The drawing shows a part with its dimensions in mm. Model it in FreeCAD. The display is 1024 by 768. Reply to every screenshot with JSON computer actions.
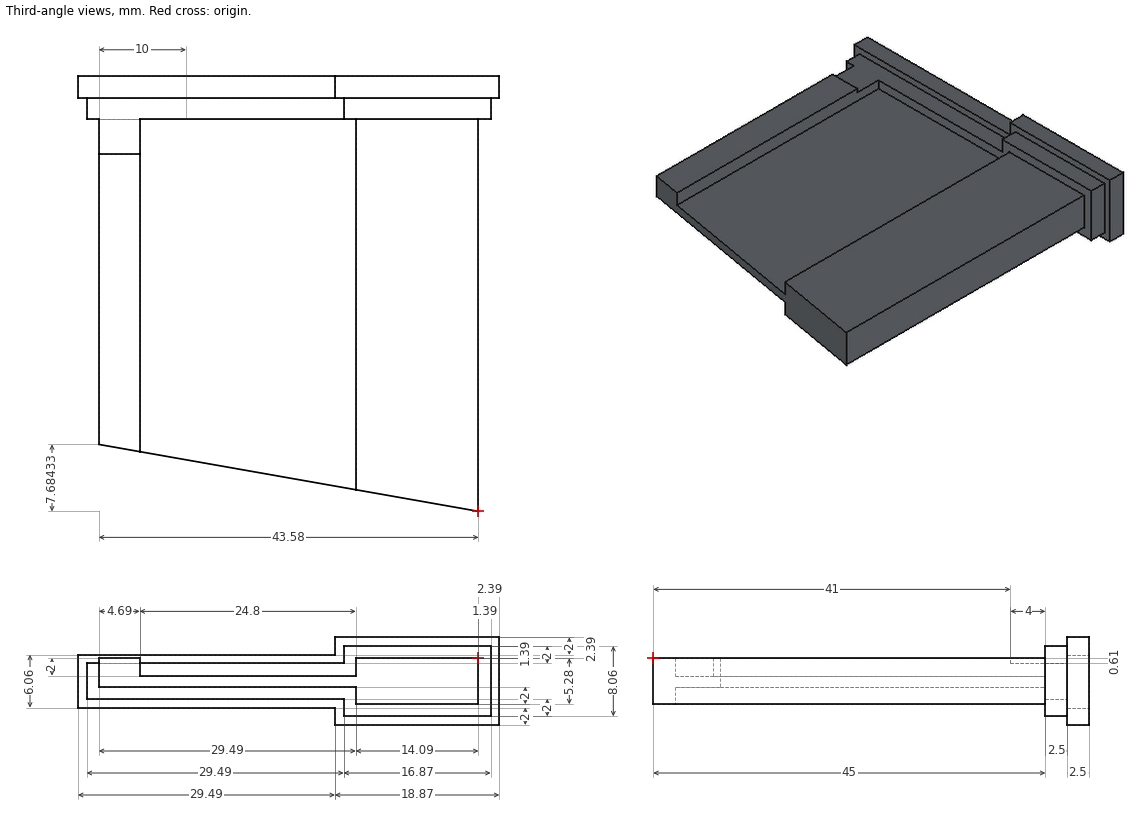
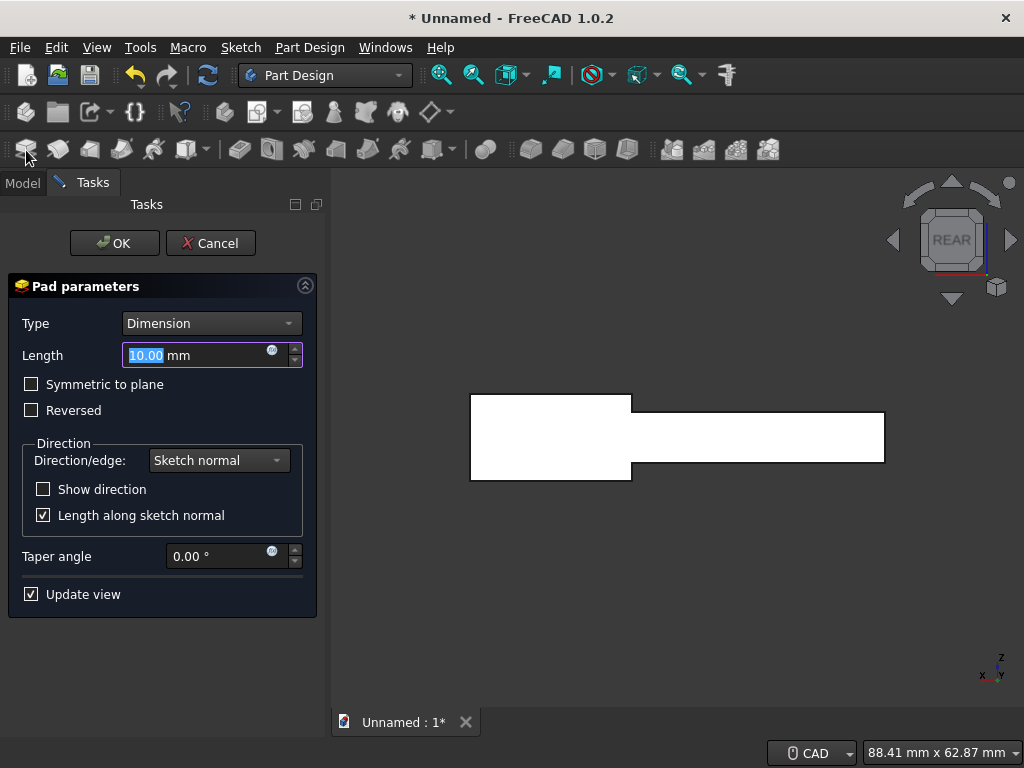
{"action": "type", "text": "2.5"}
{"action": "key", "text": "Tab"}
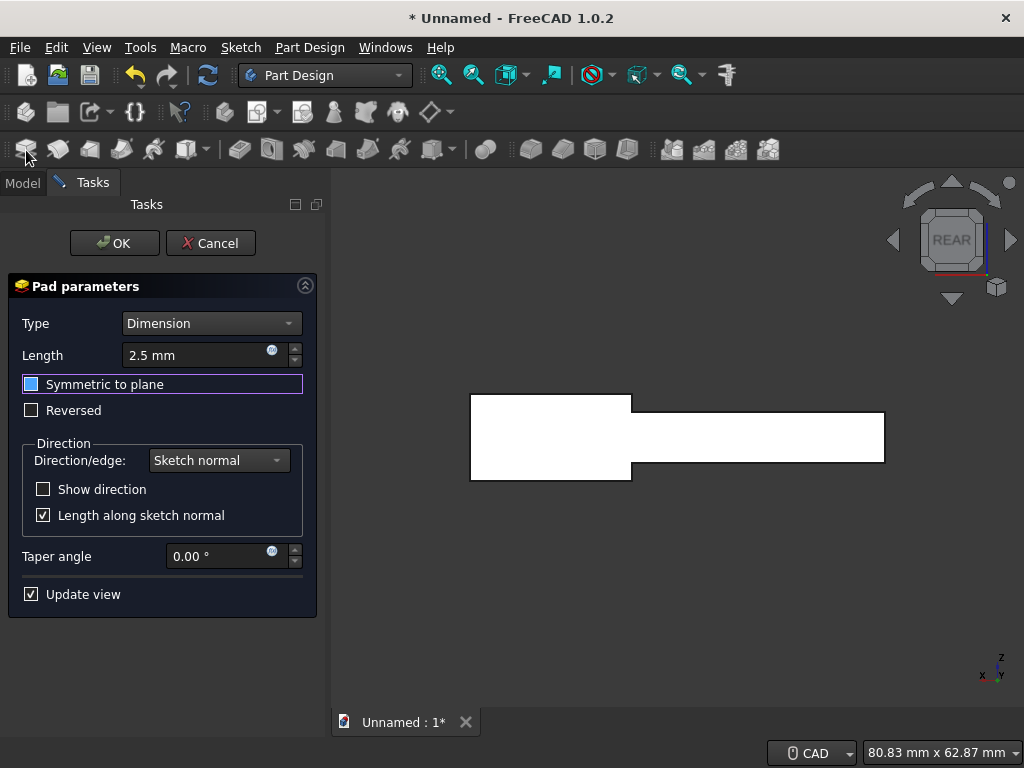
{"action": "left_click", "coordinate": [115, 243]}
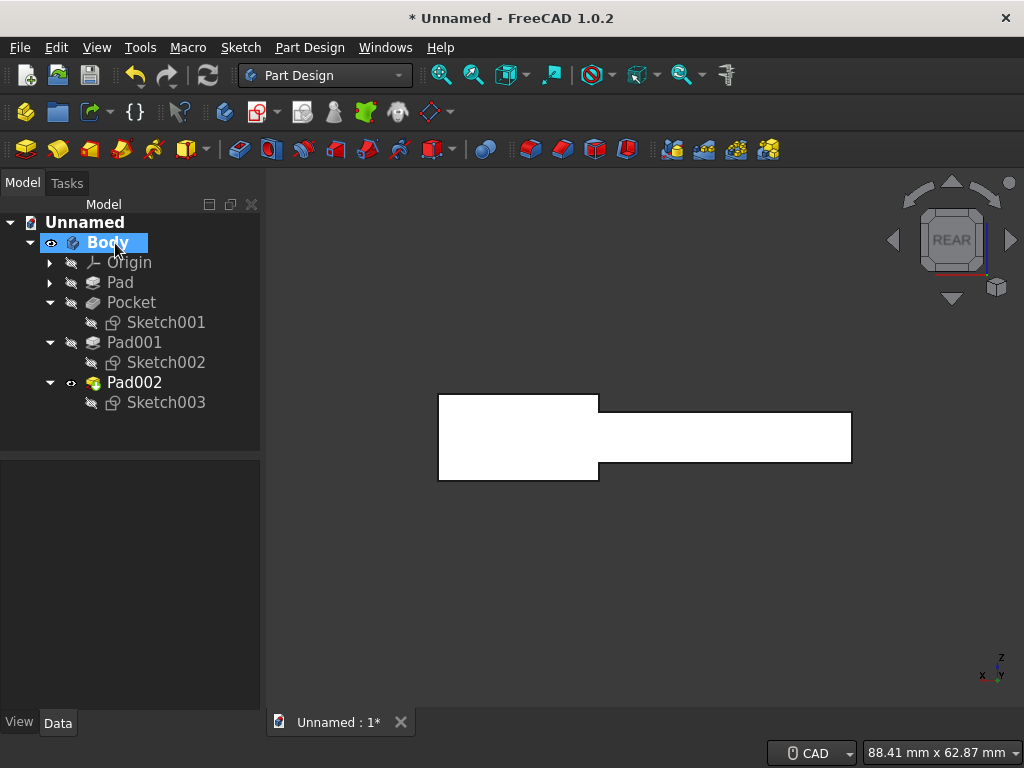
{"action": "key", "text": "6"}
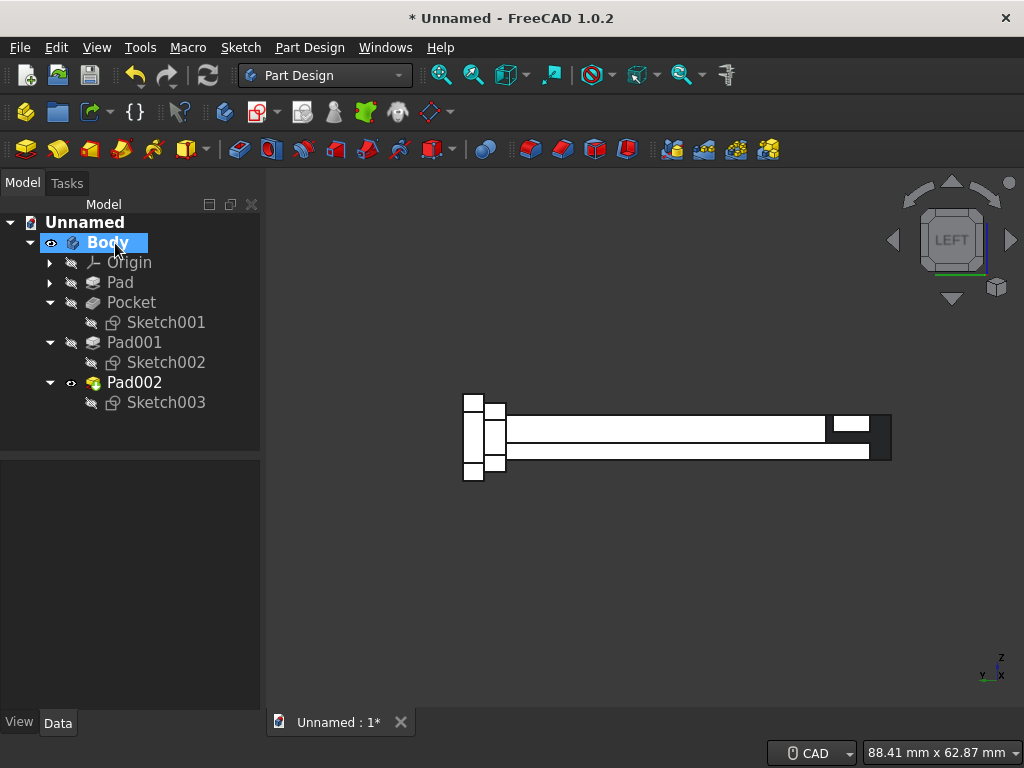
{"action": "left_click", "coordinate": [529, 428]}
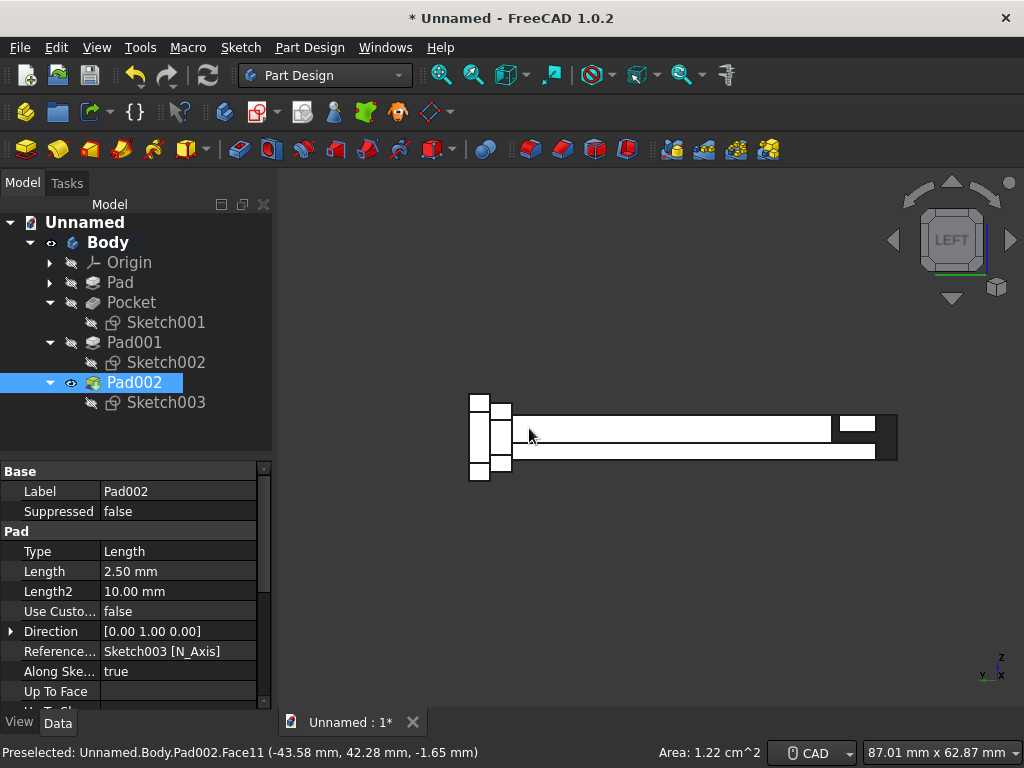
{"action": "left_click", "coordinate": [258, 112]}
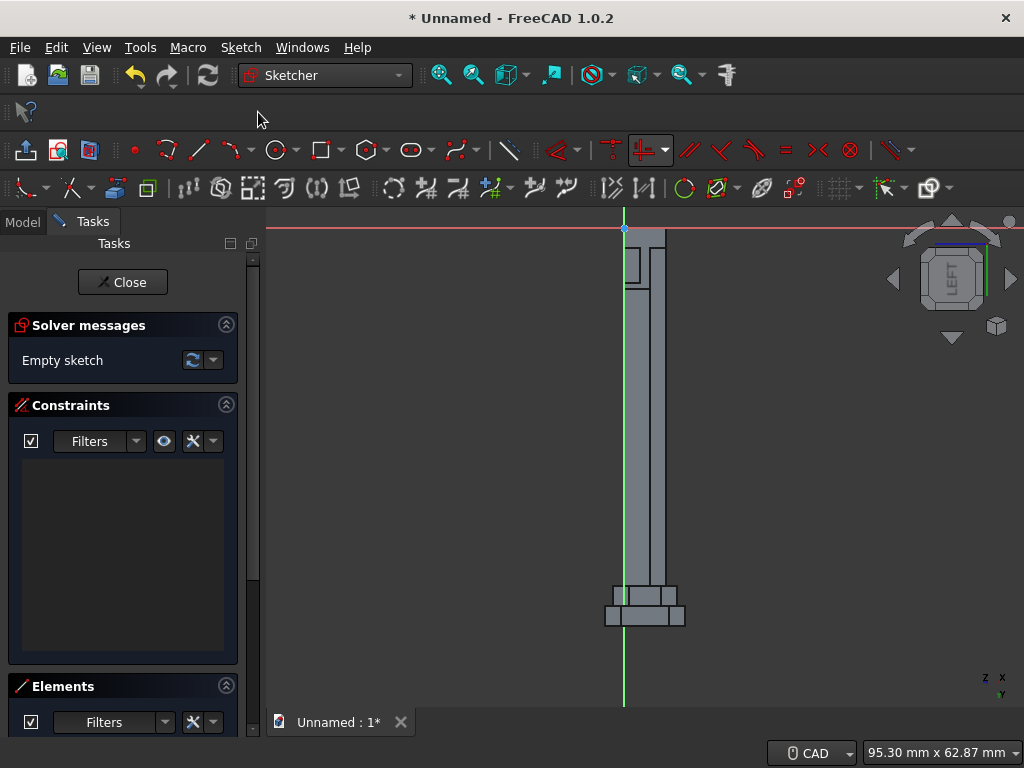
{"action": "key", "text": "q s"}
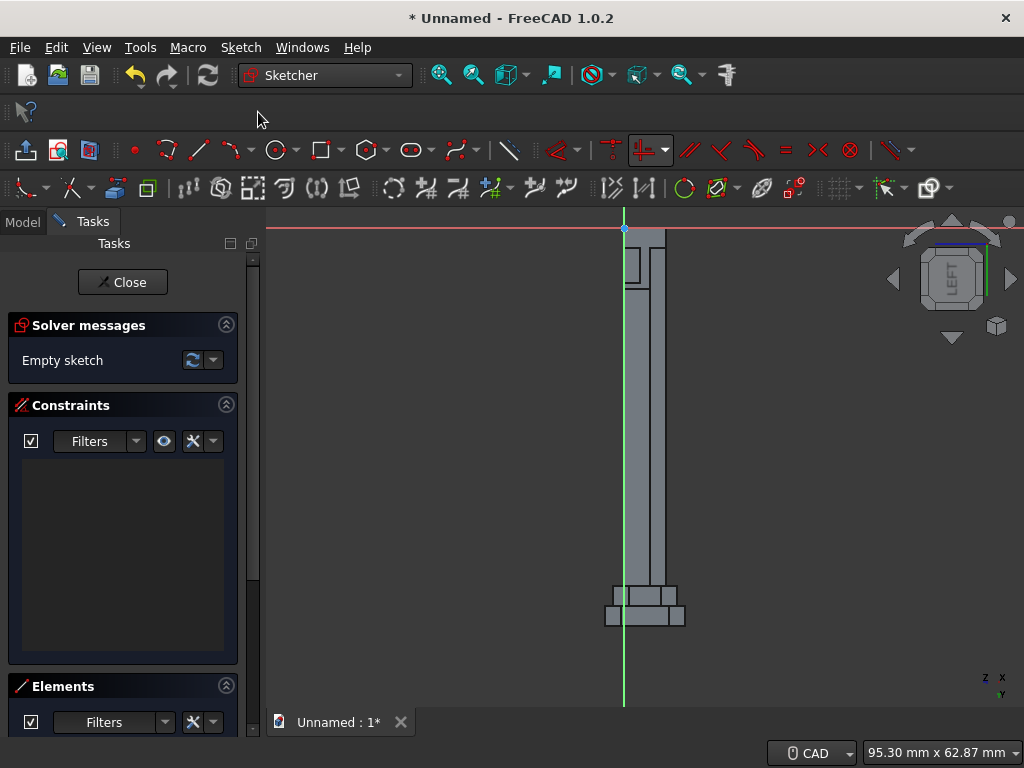
{"action": "scroll", "coordinate": [633, 584], "scroll_direction": "up", "scroll_amount": 11}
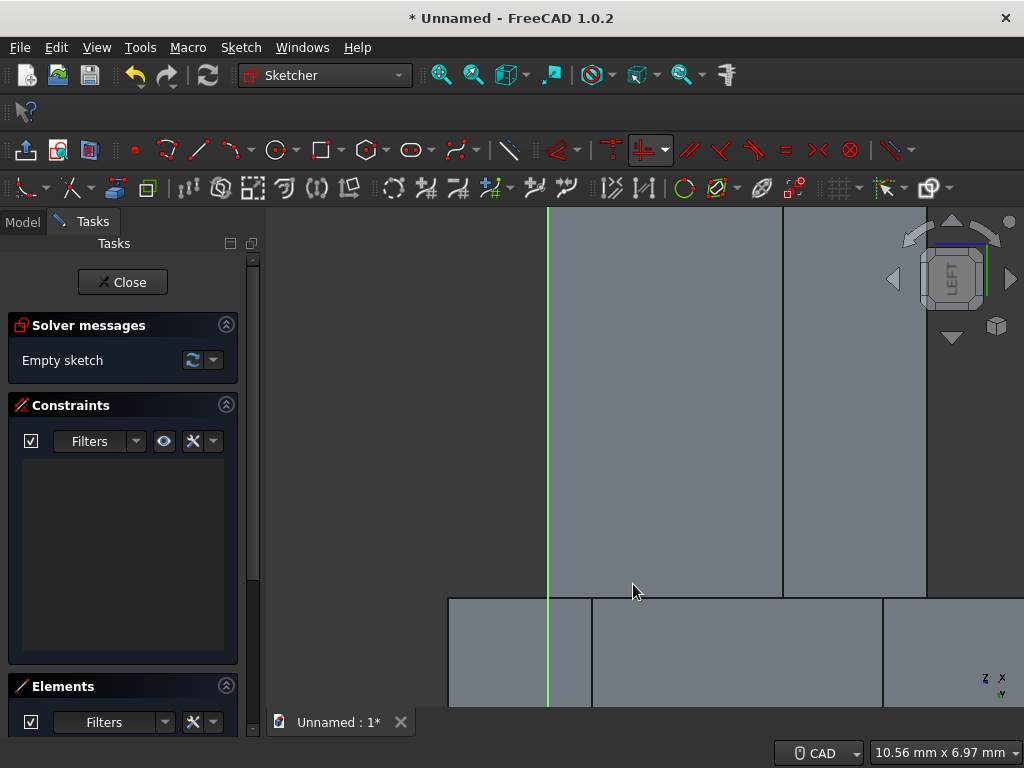
{"action": "key", "text": "g r"}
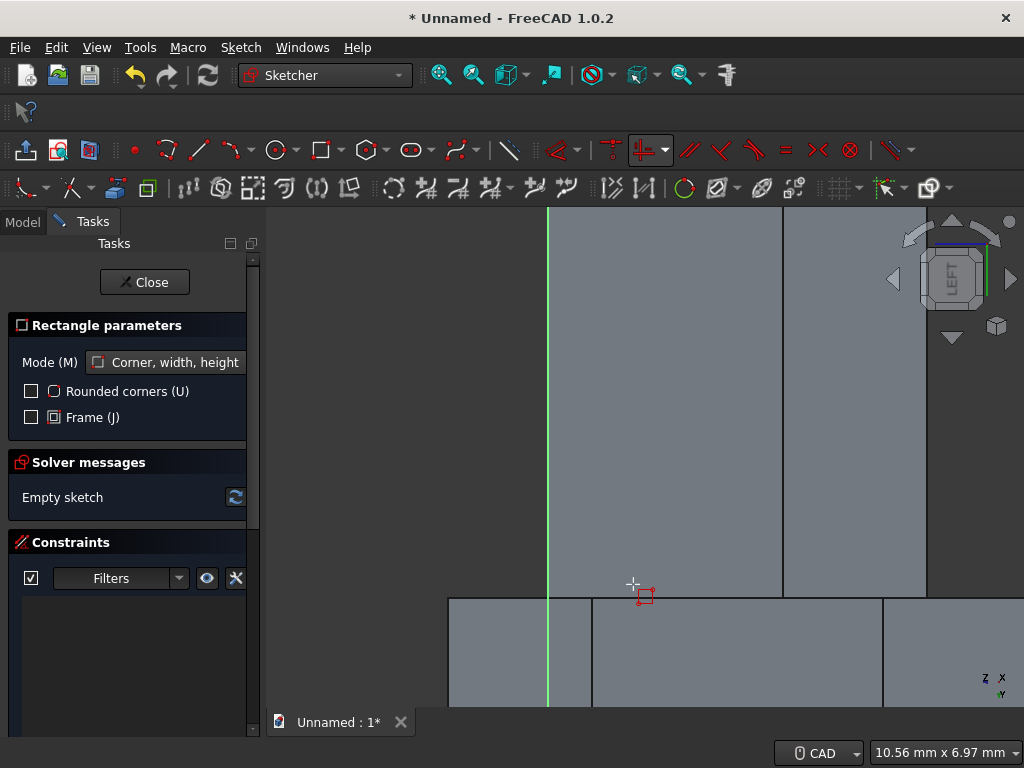
{"action": "left_click", "coordinate": [548, 311]}
{"action": "left_click", "coordinate": [592, 598]}
{"action": "key", "text": "Escape"}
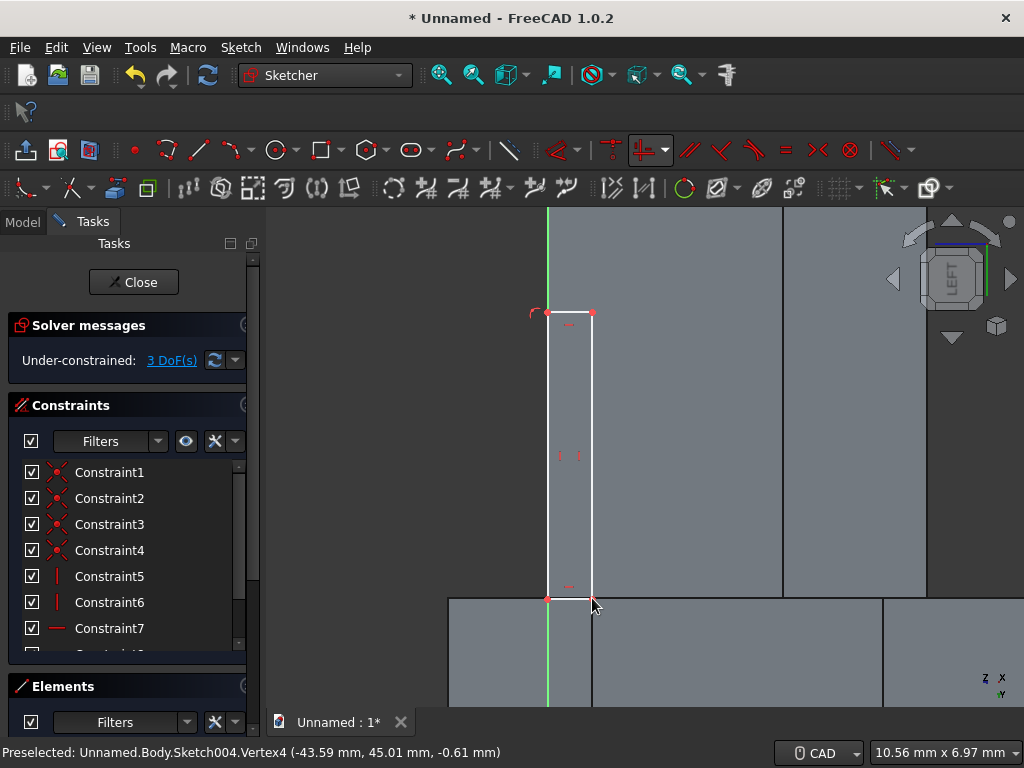
{"action": "key", "text": "d"}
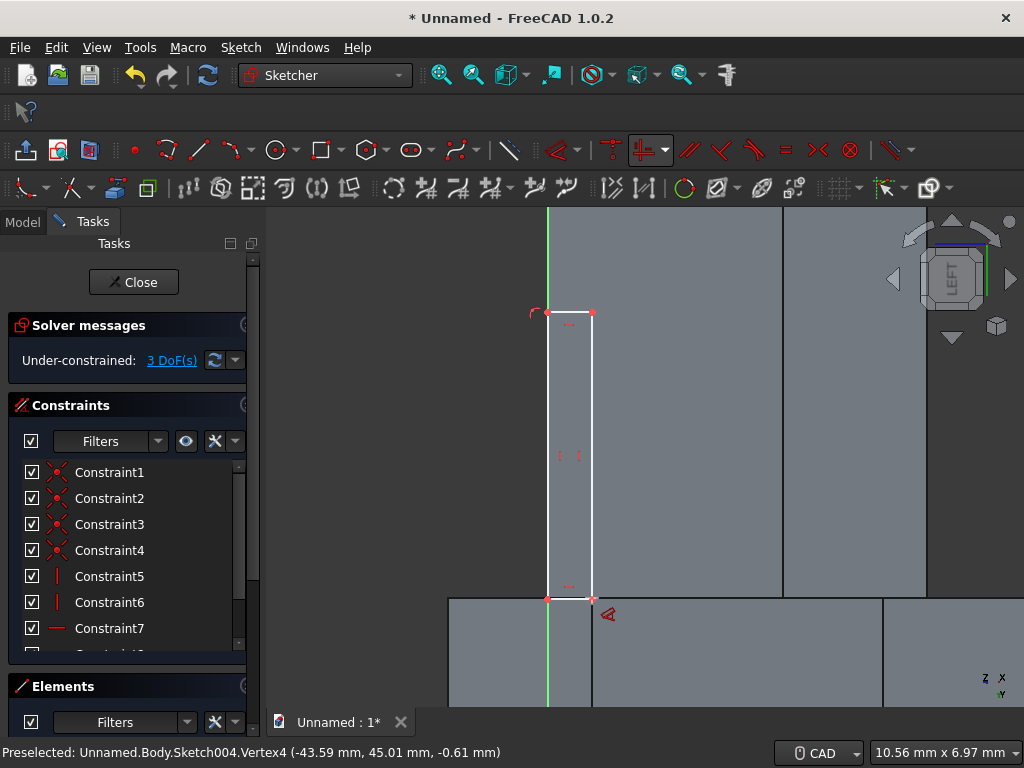
{"action": "left_click", "coordinate": [548, 398]}
{"action": "left_click", "coordinate": [514, 455]}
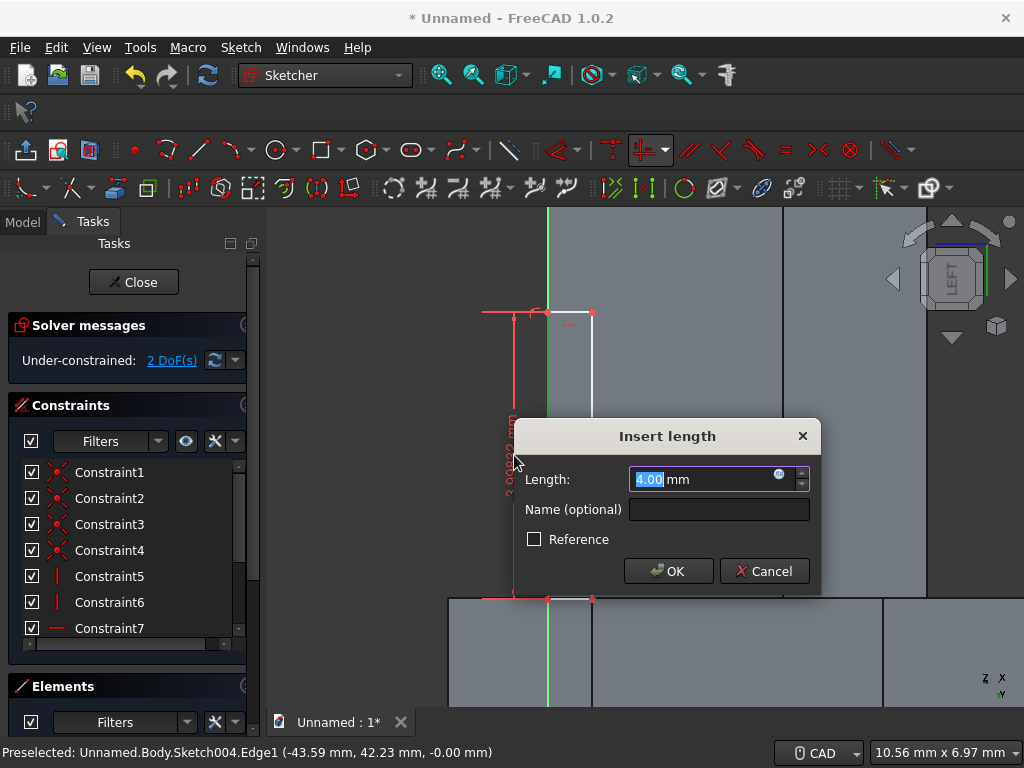
{"action": "type", "text": "4"}
{"action": "key", "text": "Return"}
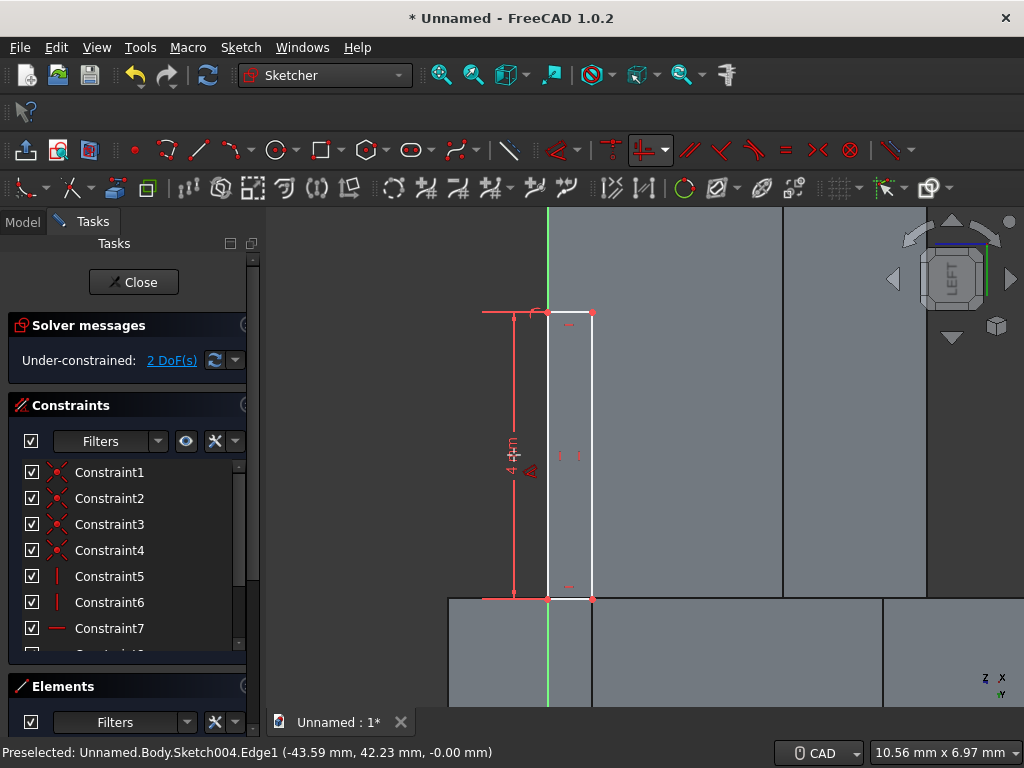
{"action": "left_click", "coordinate": [548, 312]}
{"action": "left_click", "coordinate": [514, 274]}